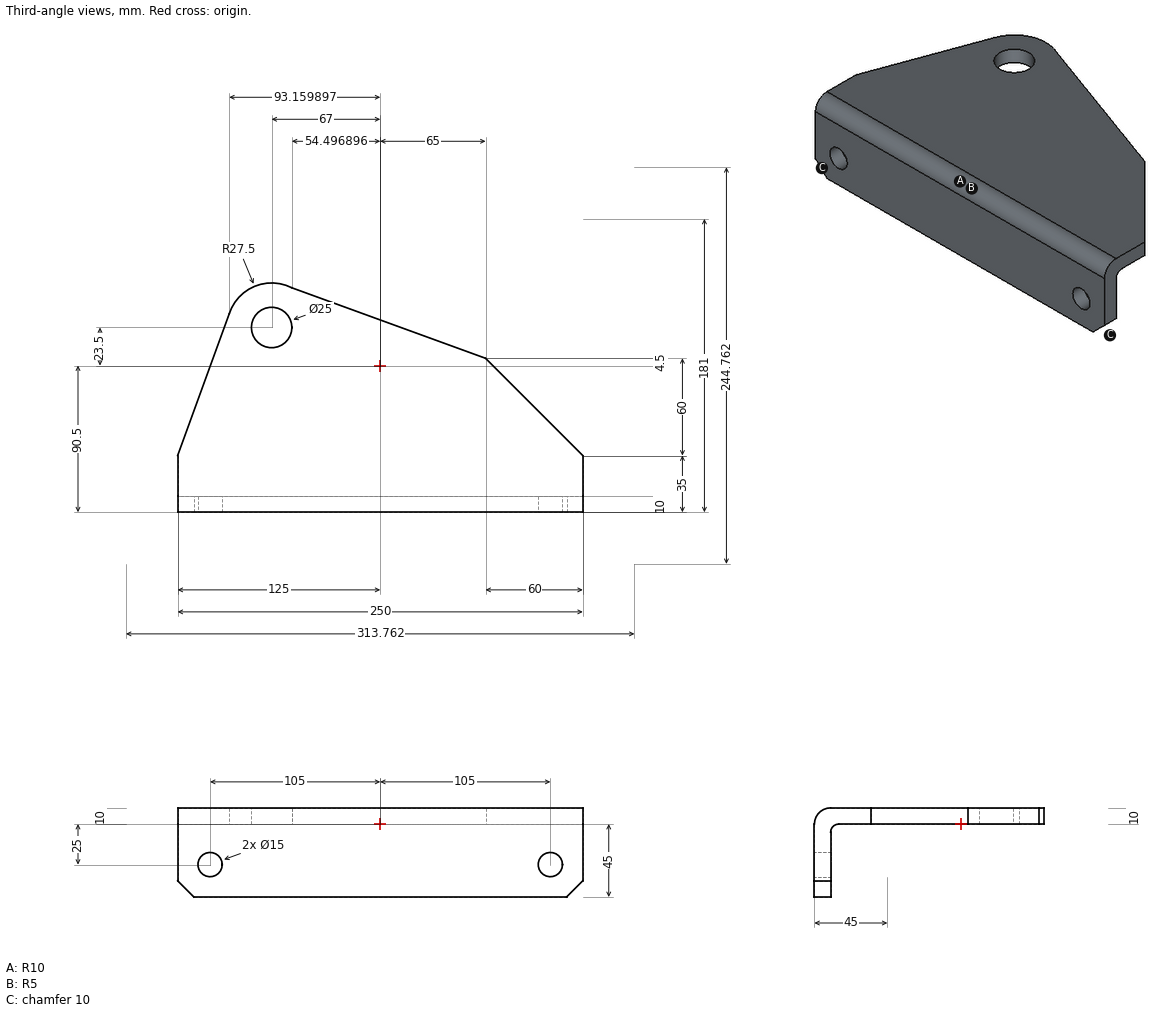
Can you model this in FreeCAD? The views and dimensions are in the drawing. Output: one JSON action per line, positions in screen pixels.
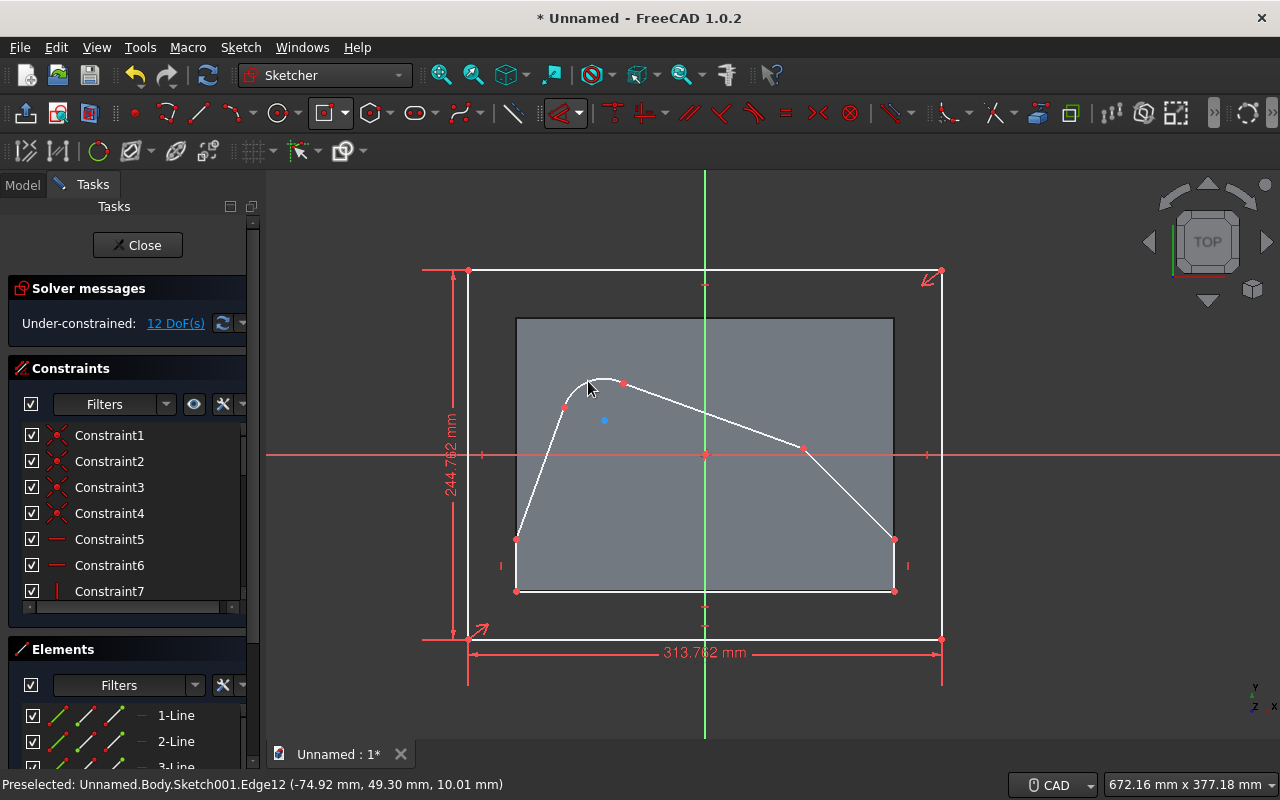
{"action": "left_click", "coordinate": [560, 114]}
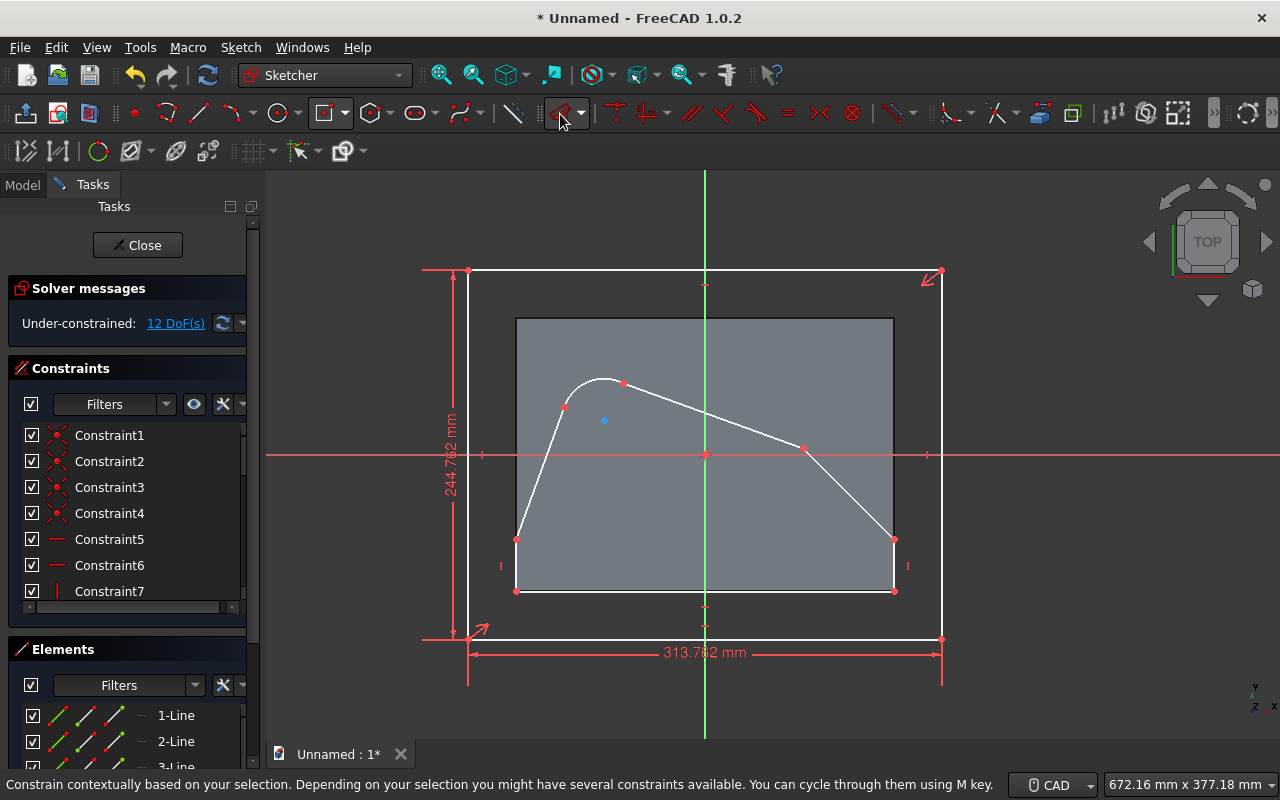
{"action": "left_click", "coordinate": [602, 379]}
{"action": "left_click", "coordinate": [600, 347]}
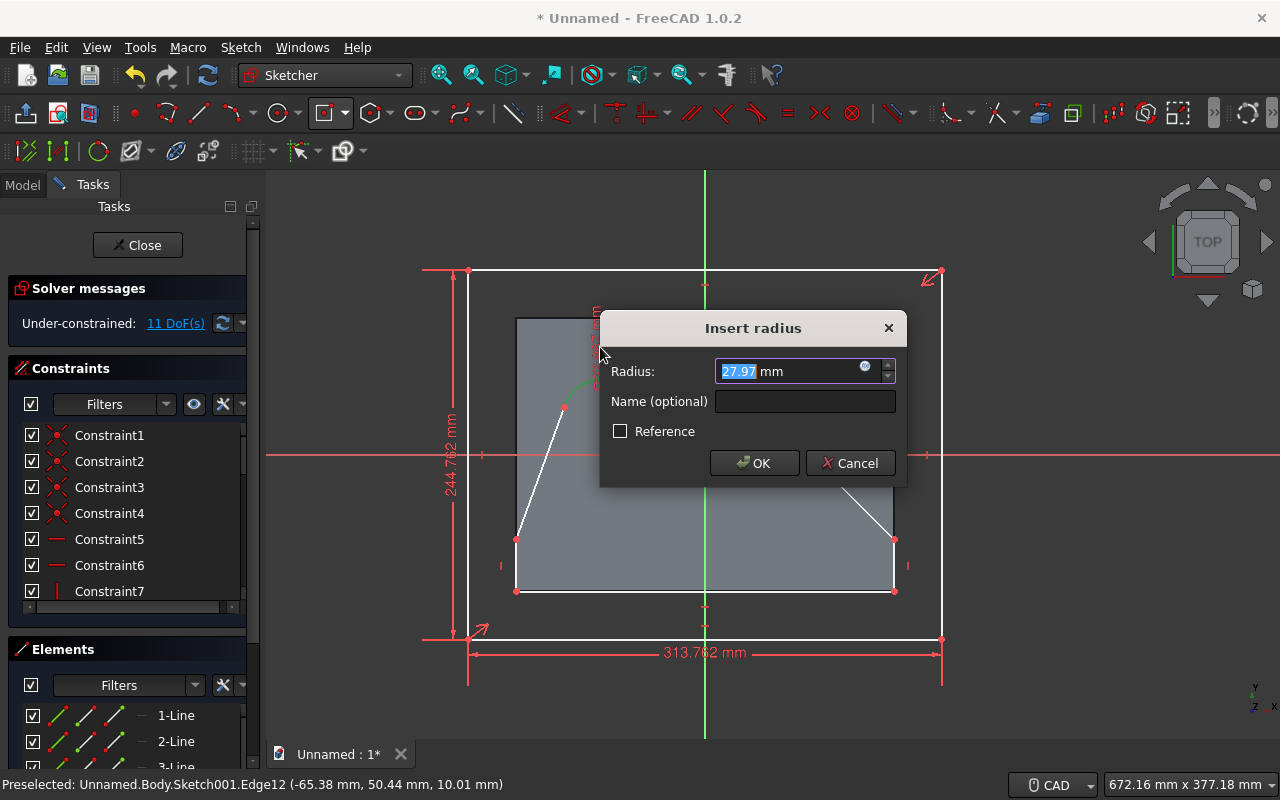
{"action": "type", "text": "27.5"}
{"action": "key", "text": "Return"}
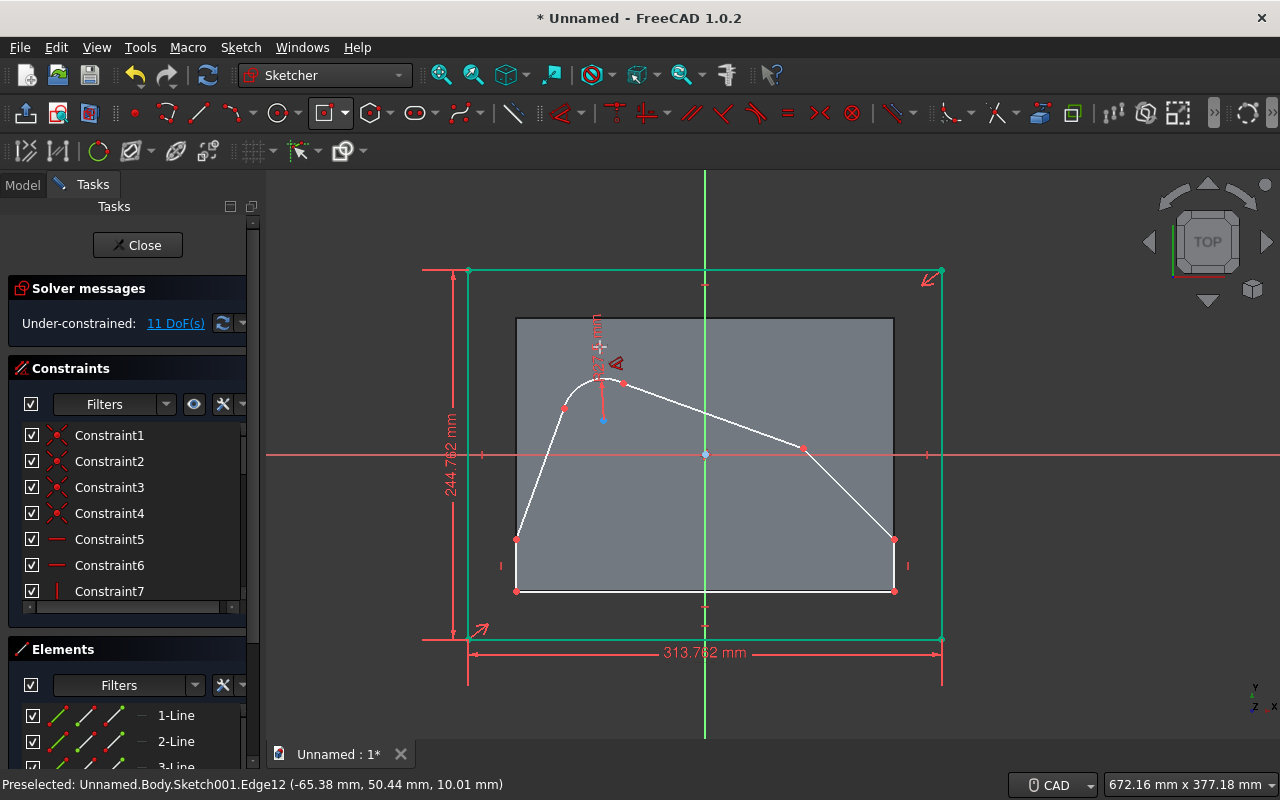
{"action": "left_click", "coordinate": [894, 556]}
{"action": "left_click", "coordinate": [928, 566]}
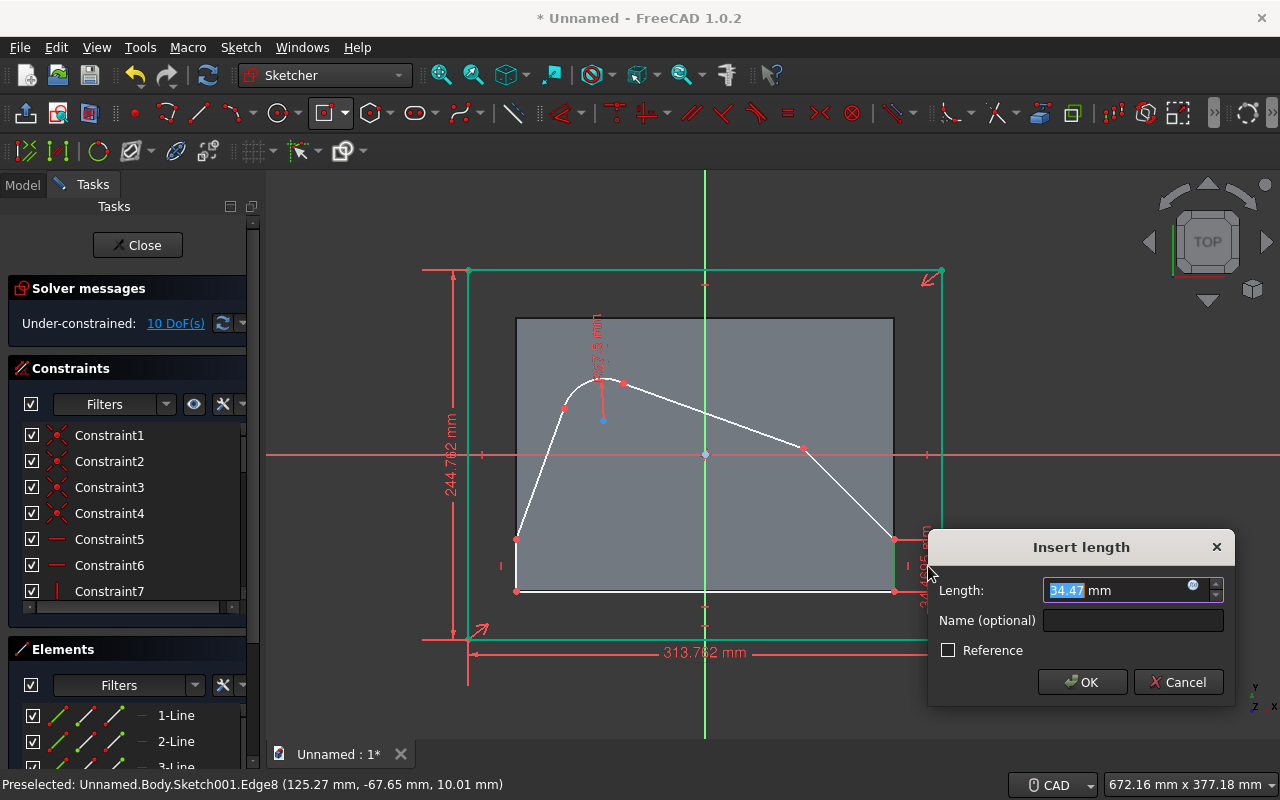
{"action": "type", "text": "35"}
{"action": "key", "text": "Return"}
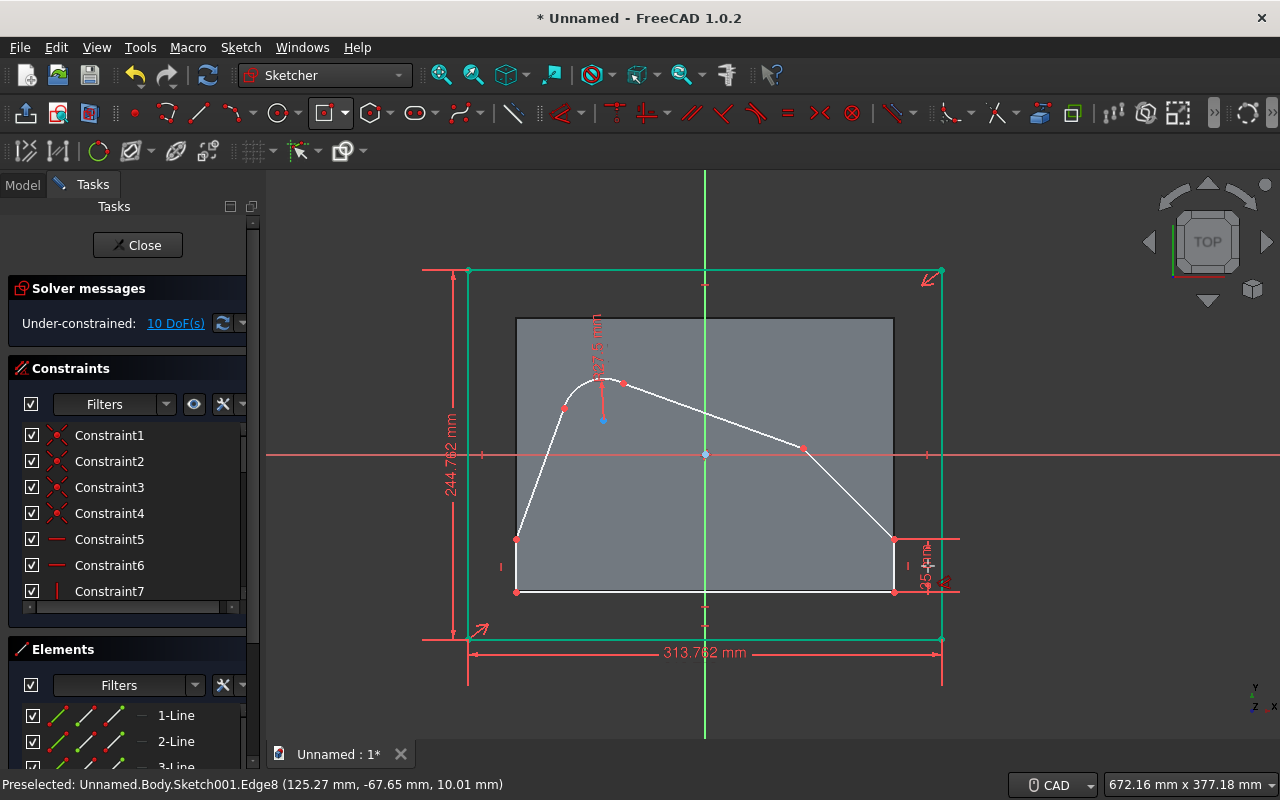
{"action": "left_click", "coordinate": [516, 577]}
{"action": "left_click", "coordinate": [482, 566]}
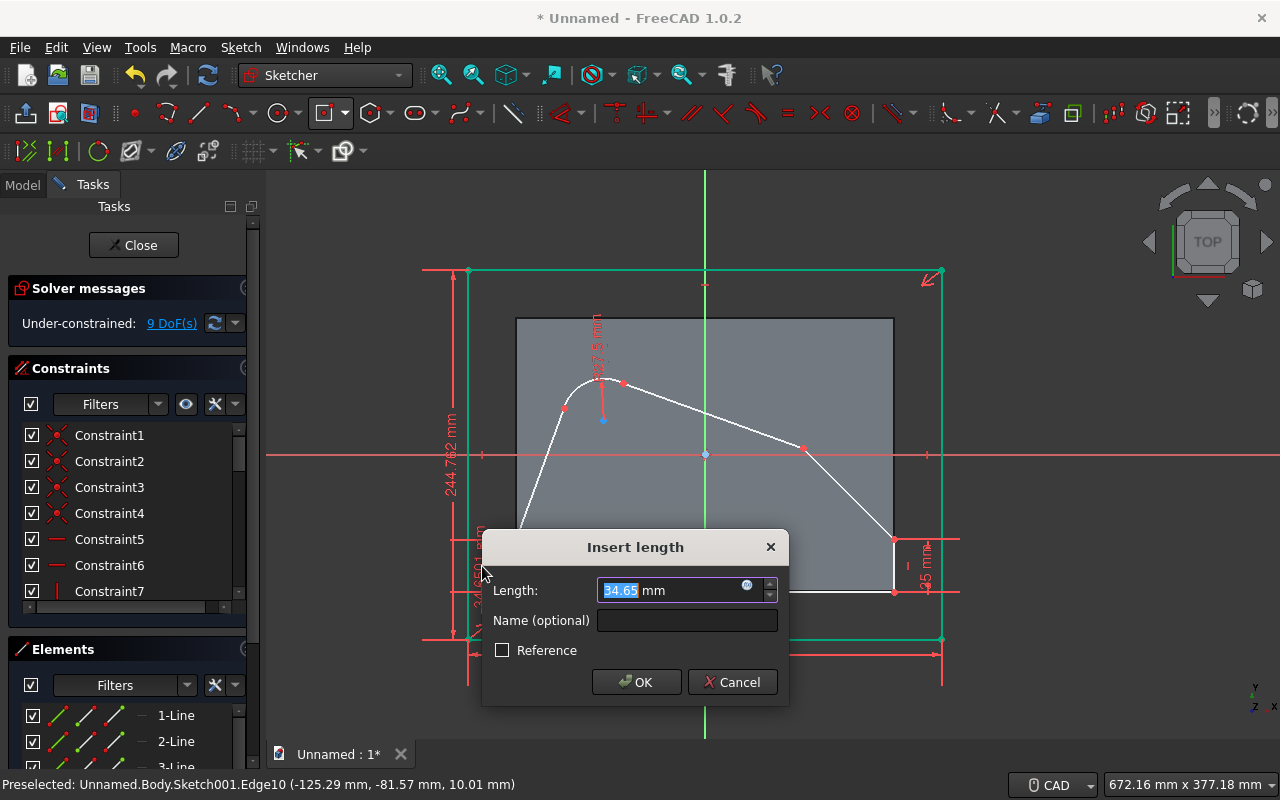
{"action": "type", "text": "35"}
{"action": "key", "text": "Return"}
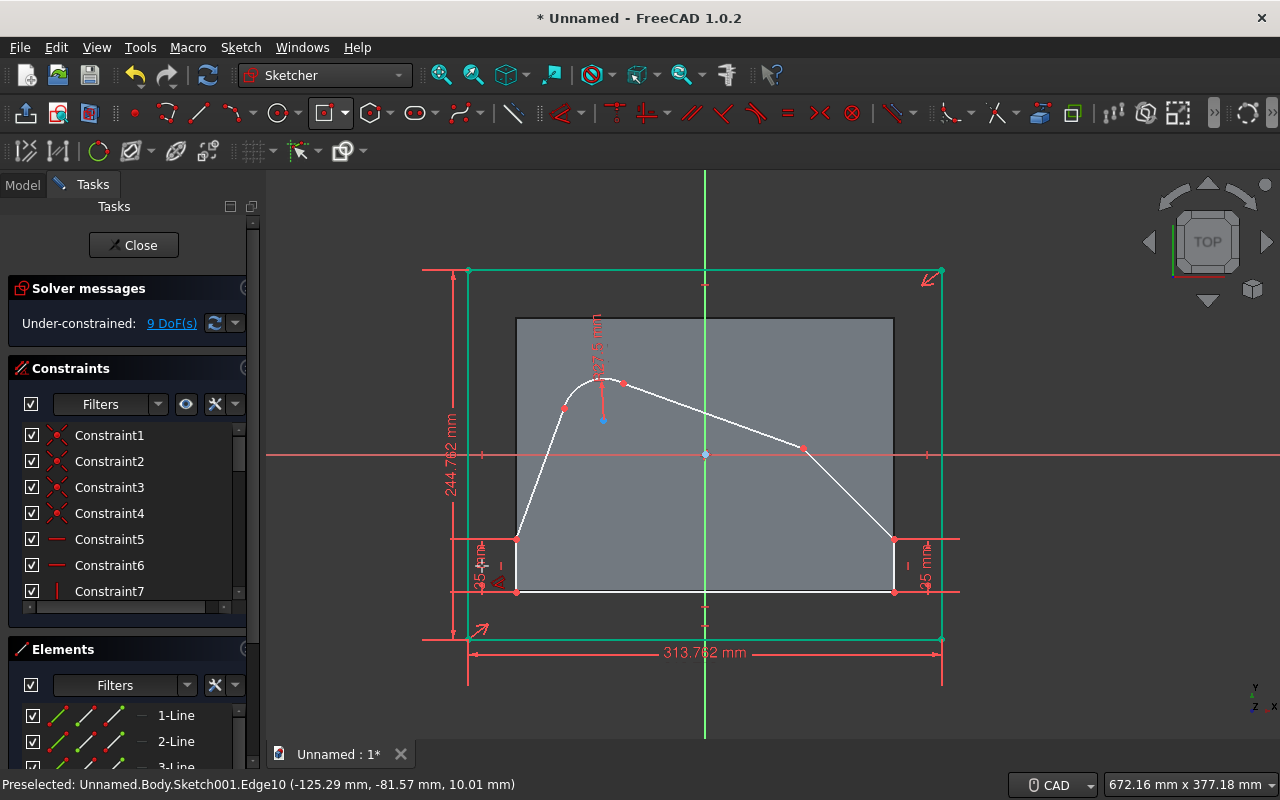
{"action": "left_click", "coordinate": [781, 592]}
{"action": "left_click", "coordinate": [618, 626]}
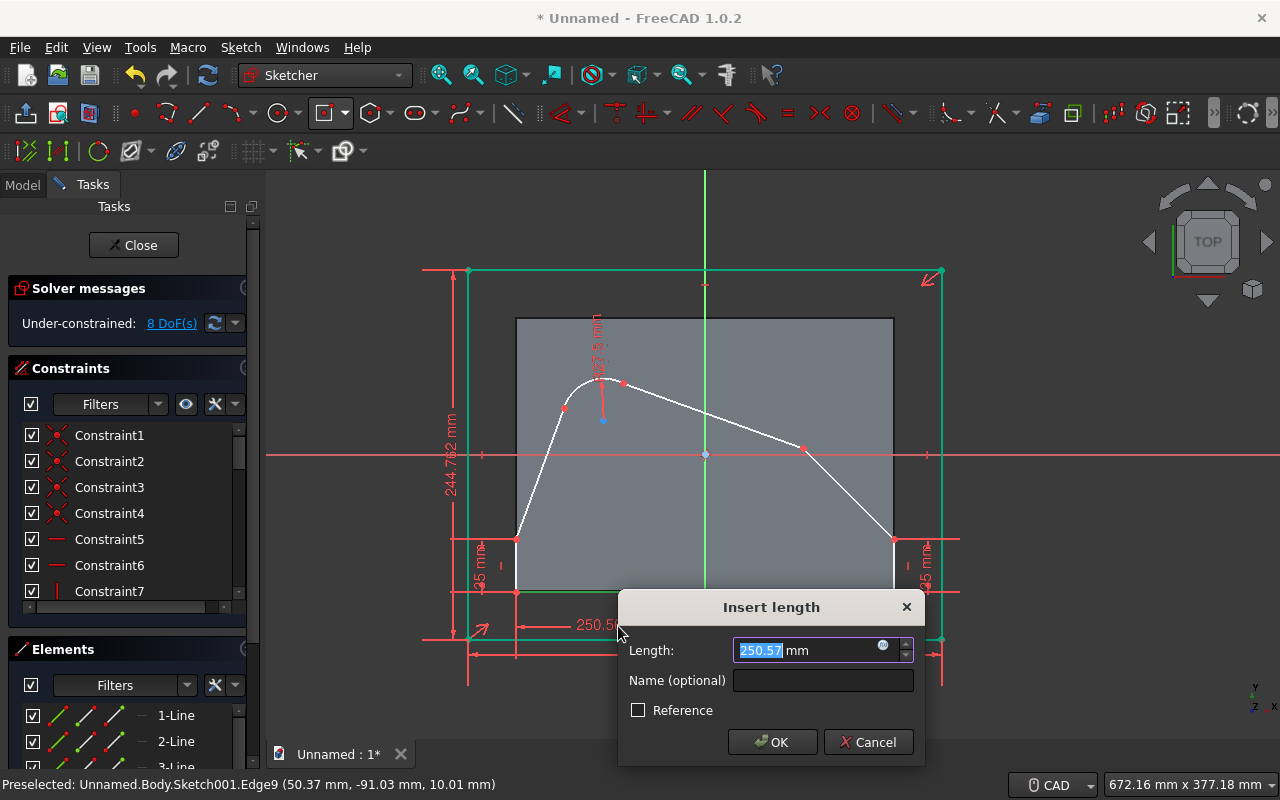
{"action": "type", "text": "250"}
{"action": "key", "text": "Return"}